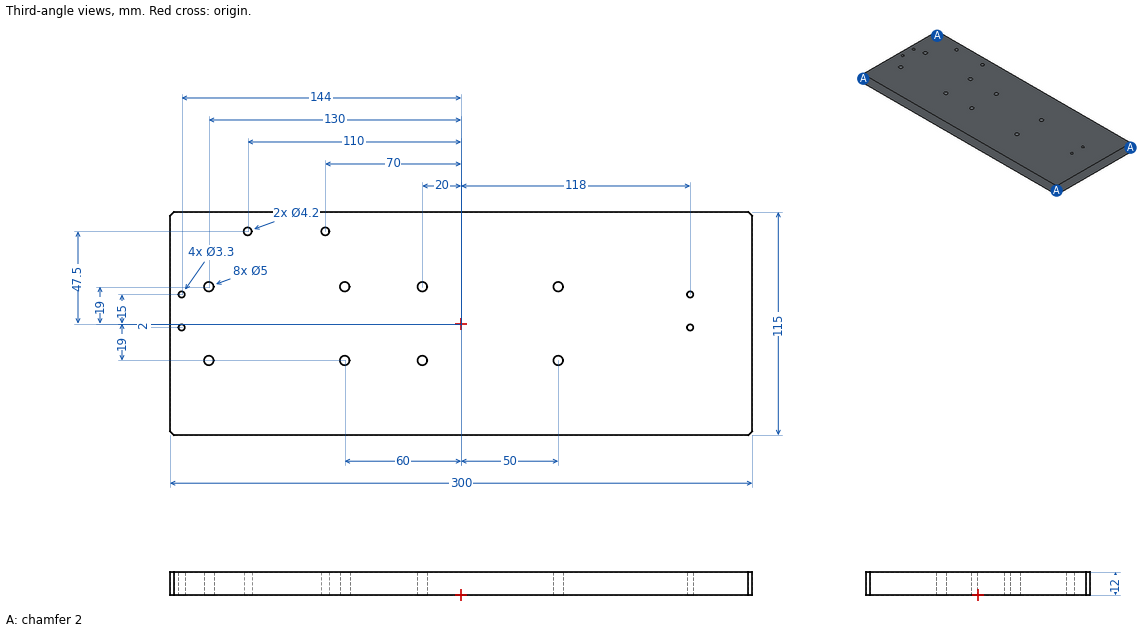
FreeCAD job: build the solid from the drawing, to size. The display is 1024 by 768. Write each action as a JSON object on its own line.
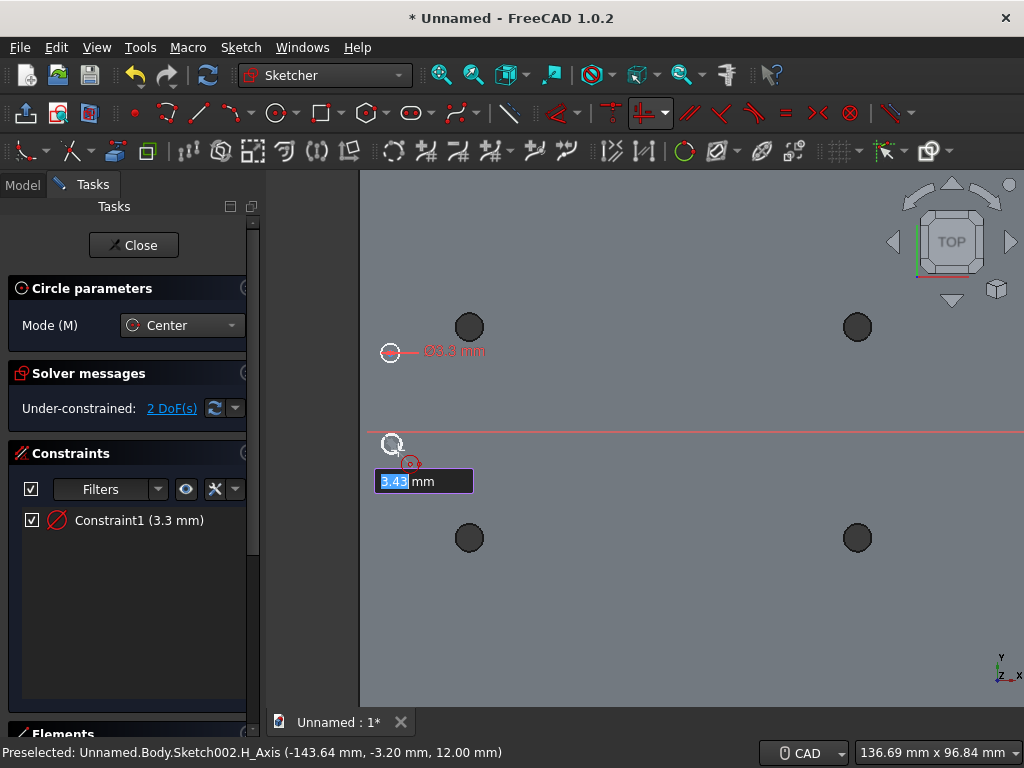
{"action": "type", "text": "3.3"}
{"action": "key", "text": "Return"}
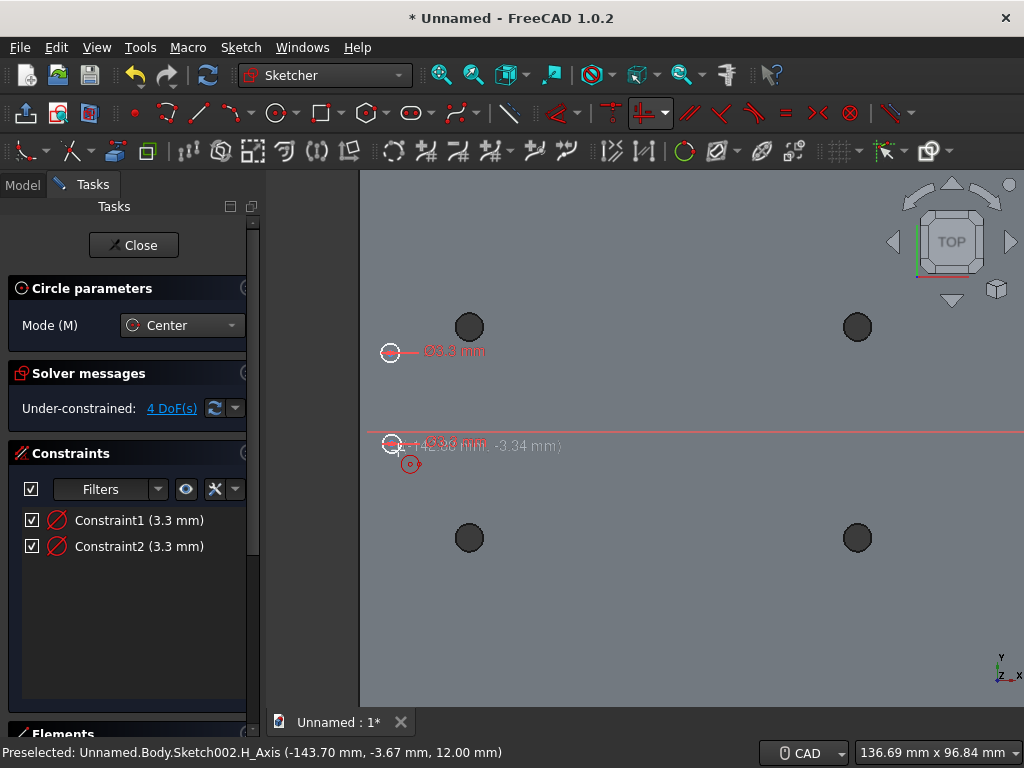
{"action": "scroll", "coordinate": [399, 452], "scroll_direction": "down", "scroll_amount": 7}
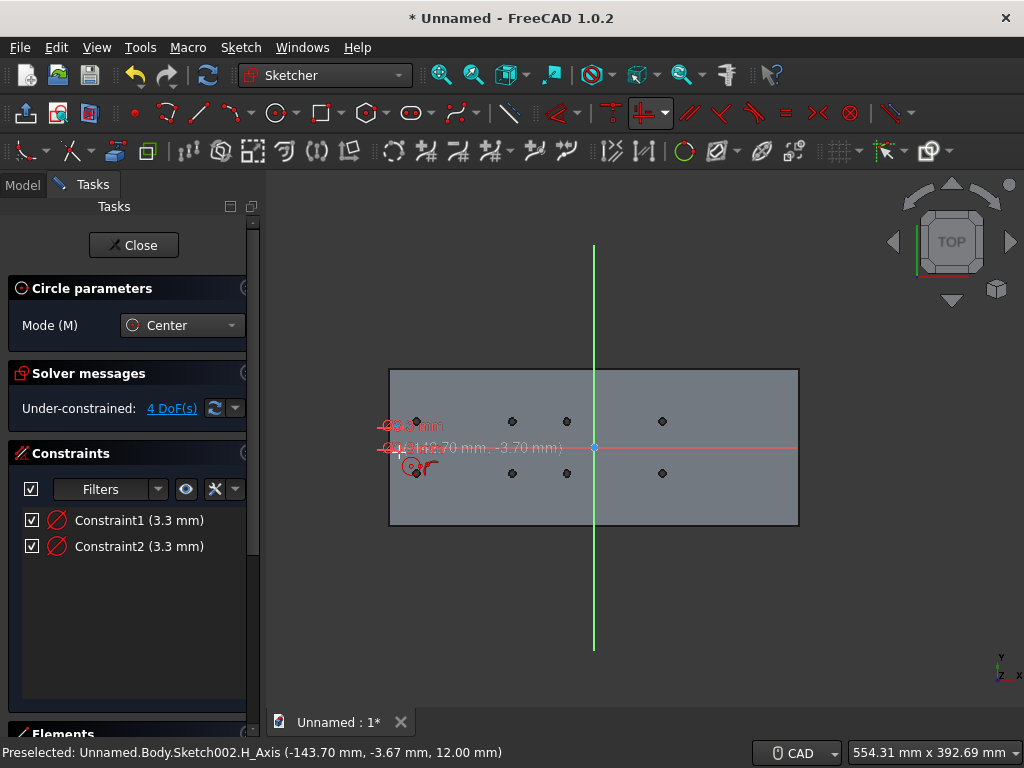
{"action": "scroll", "coordinate": [756, 427], "scroll_direction": "up", "scroll_amount": 12}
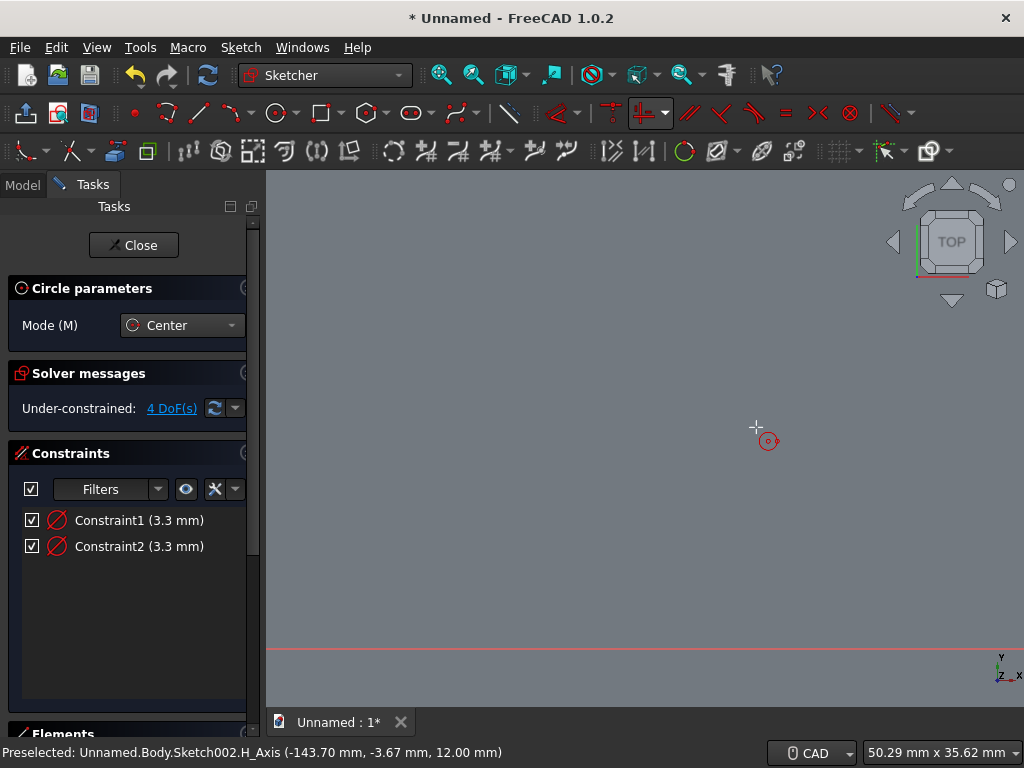
{"action": "scroll", "coordinate": [757, 427], "scroll_direction": "down", "scroll_amount": 12}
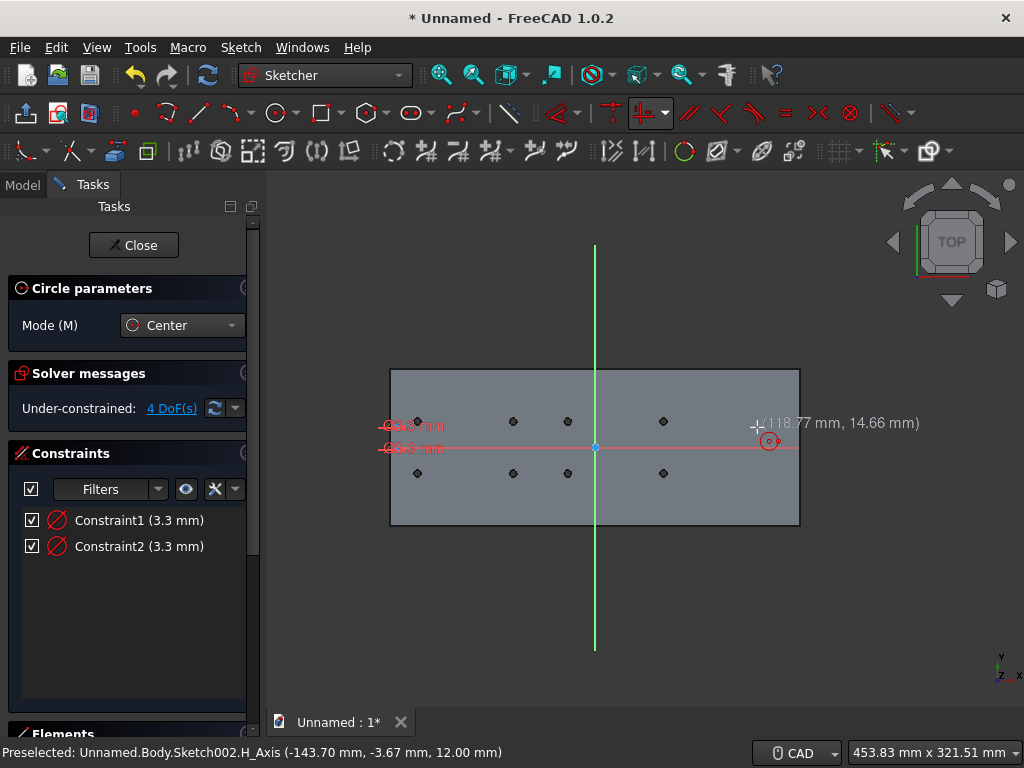
{"action": "left_click", "coordinate": [757, 427]}
{"action": "mouse_move", "coordinate": [758, 425]}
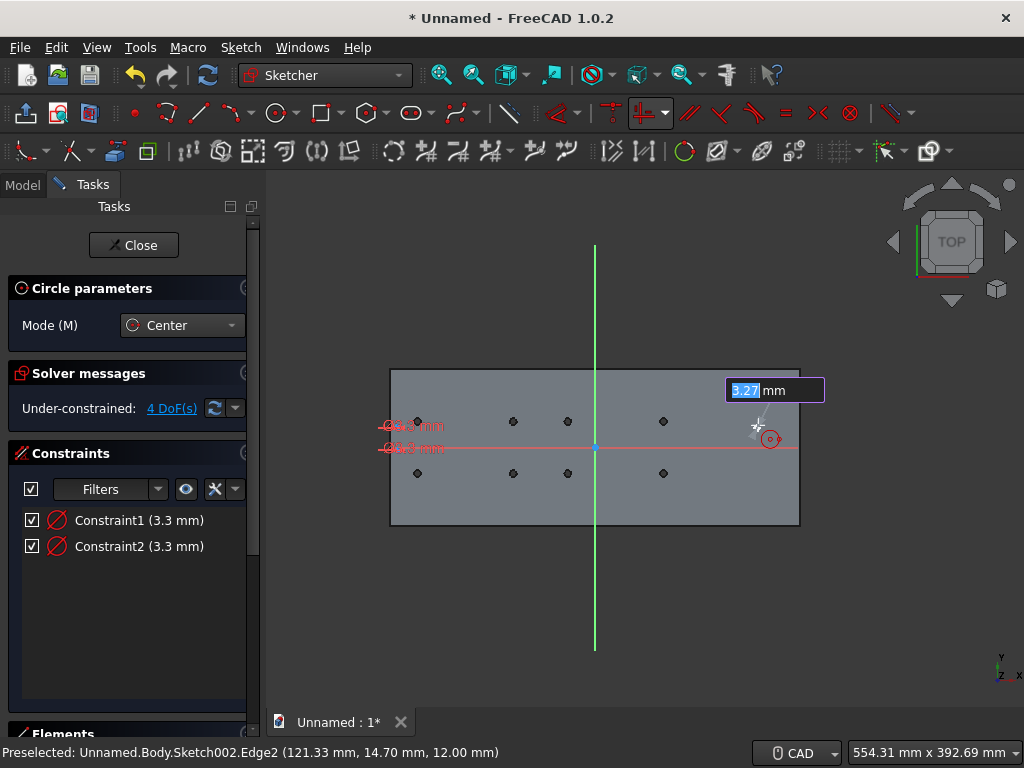
{"action": "type", "text": "3.3"}
{"action": "key", "text": "Return"}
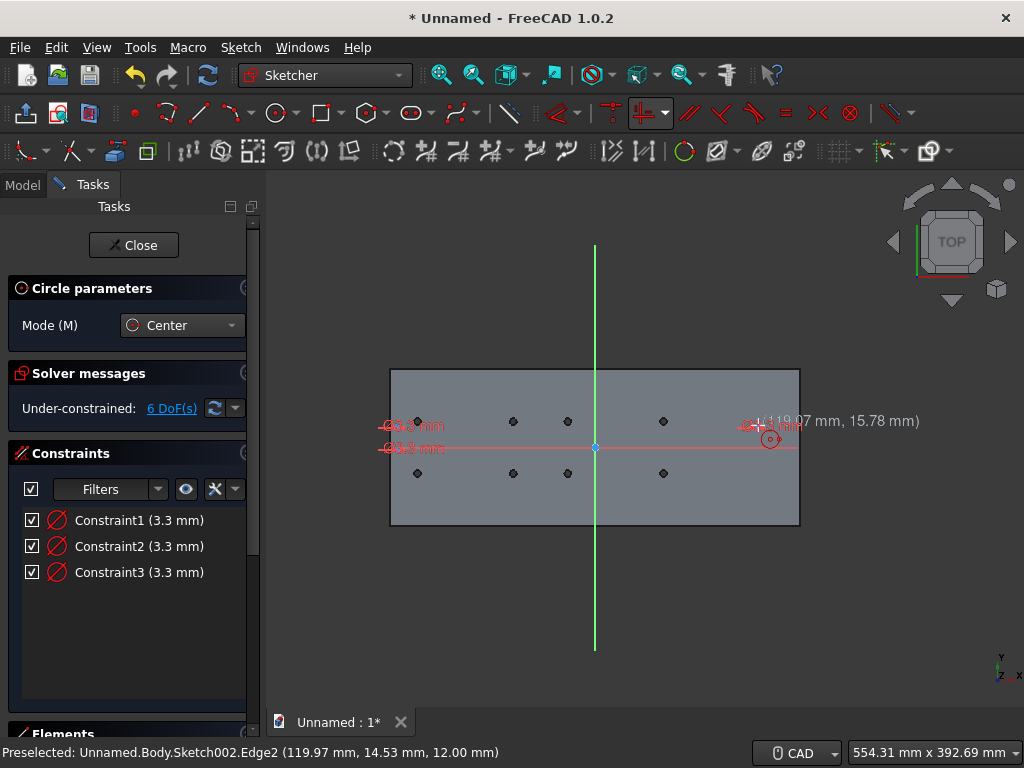
{"action": "scroll", "coordinate": [757, 450], "scroll_direction": "up", "scroll_amount": 12}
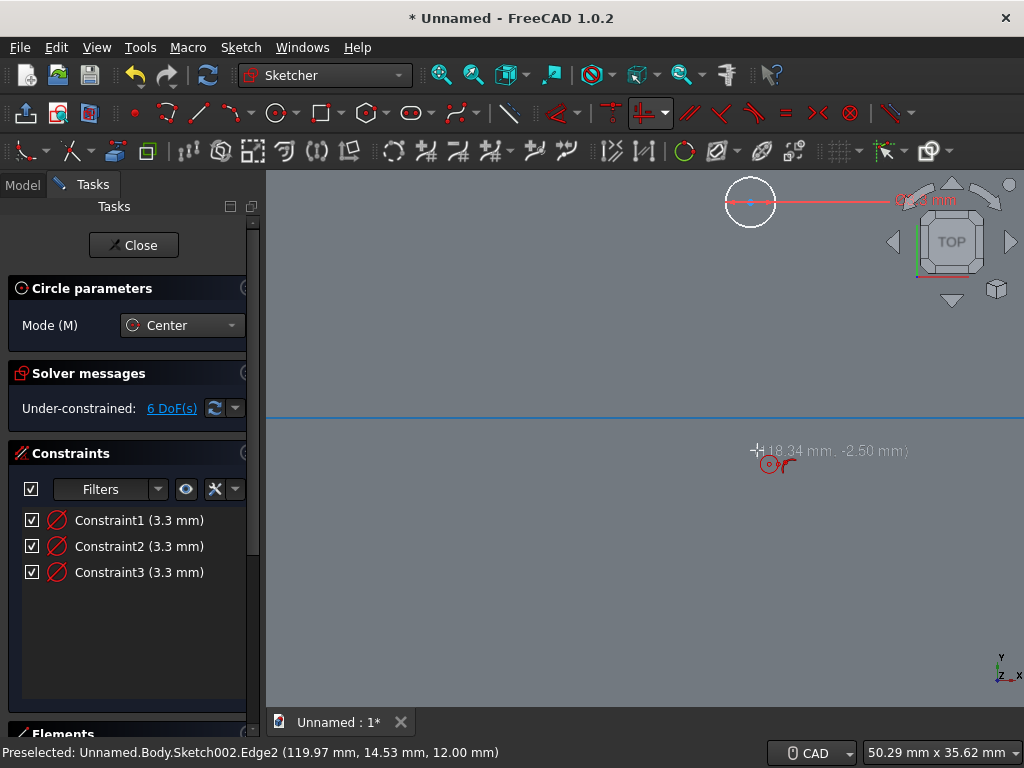
{"action": "left_click", "coordinate": [745, 448]}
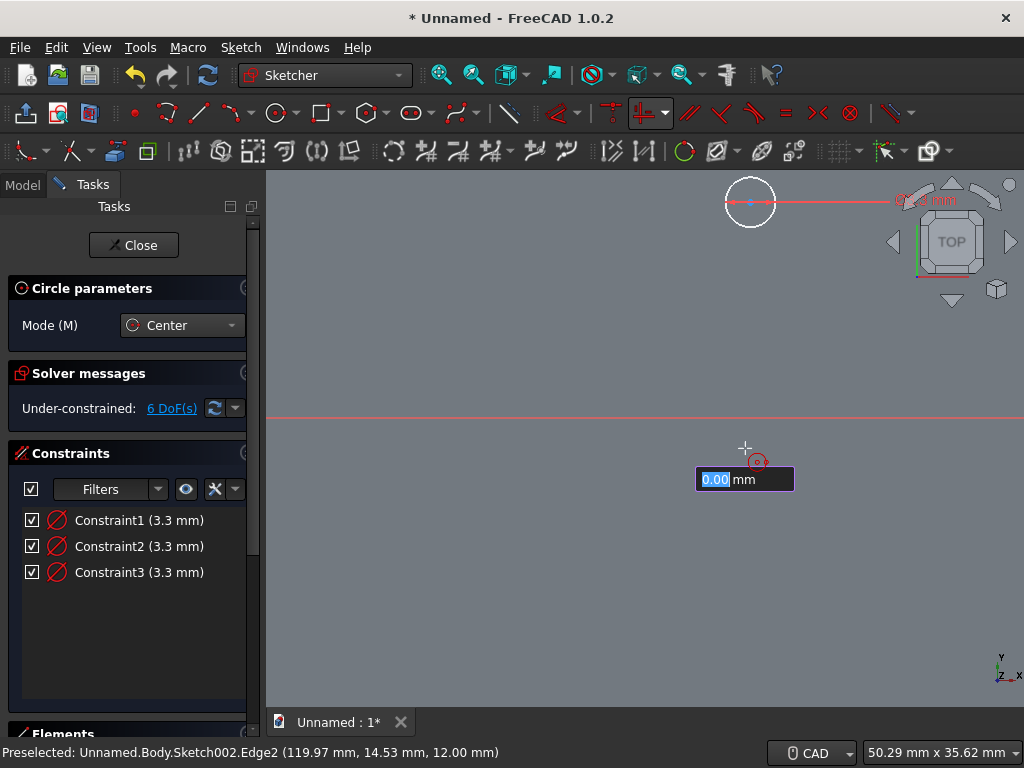
{"action": "scroll", "coordinate": [757, 450], "scroll_direction": "down", "scroll_amount": 12}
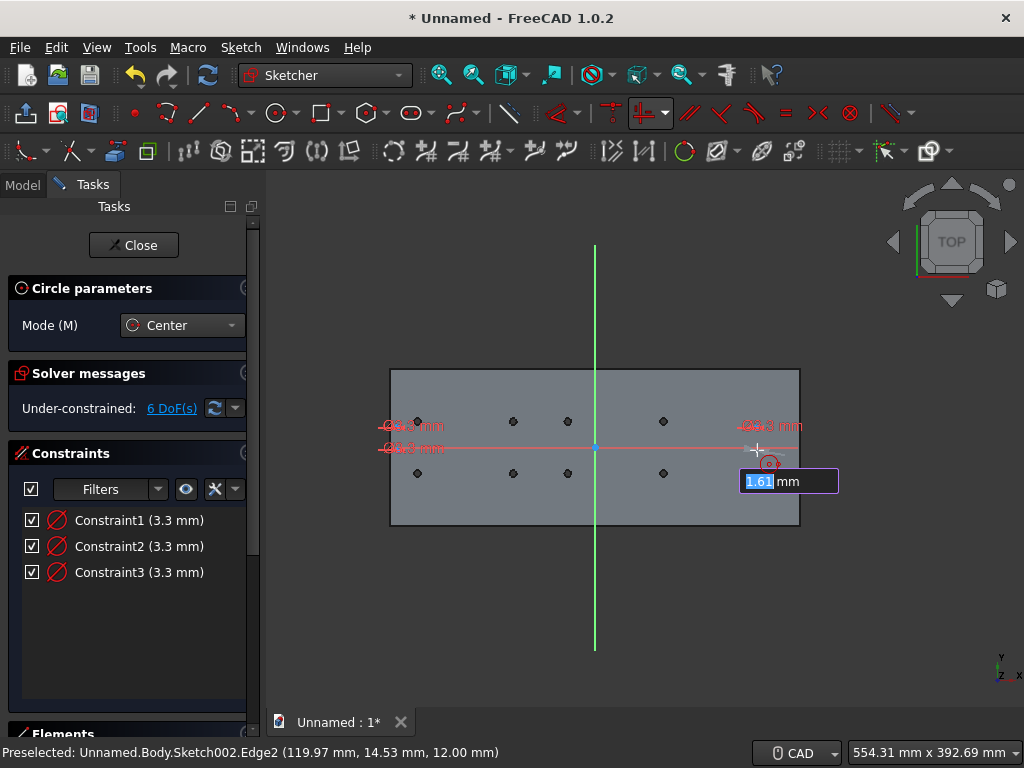
{"action": "scroll", "coordinate": [758, 452], "scroll_direction": "up", "scroll_amount": 7}
{"action": "mouse_move", "coordinate": [757, 450]}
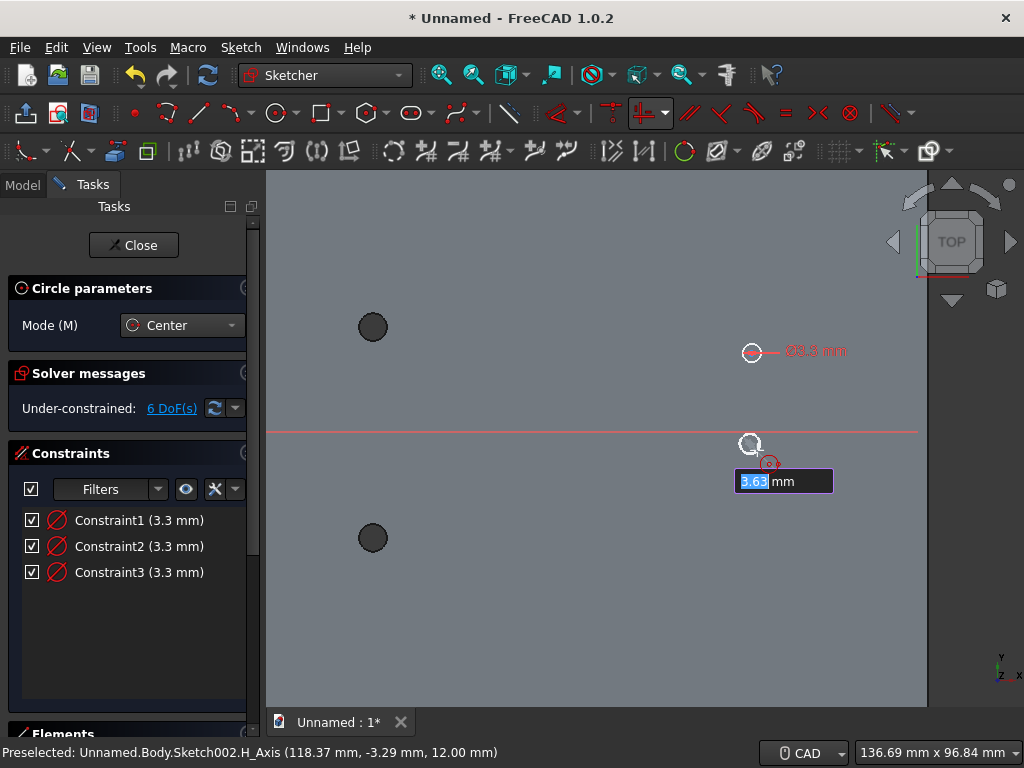
{"action": "type", "text": "3.3"}
{"action": "key", "text": "Return"}
{"action": "key", "text": "Escape"}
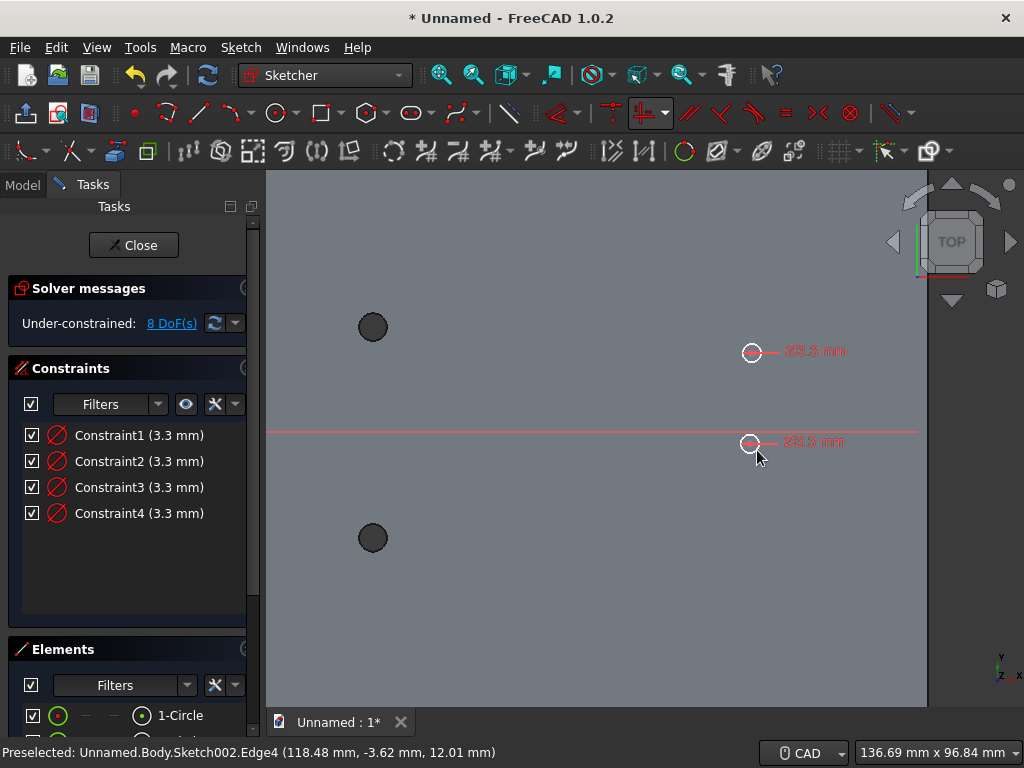
{"action": "scroll", "coordinate": [757, 452], "scroll_direction": "down", "scroll_amount": 7}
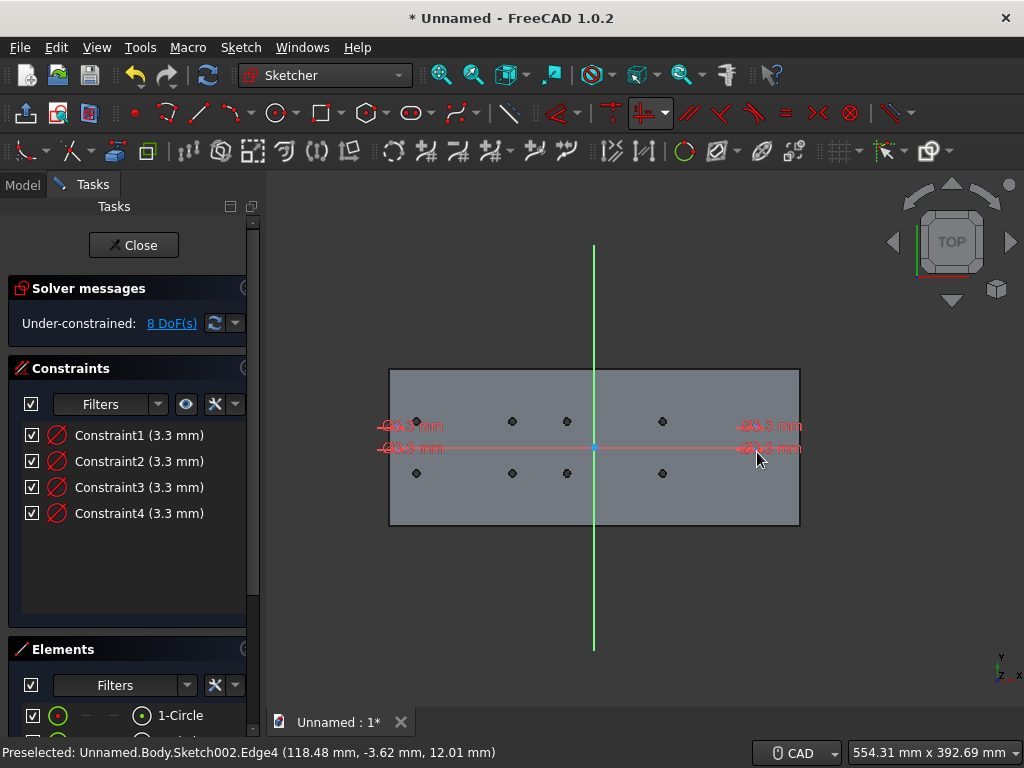
{"action": "left_click", "coordinate": [397, 428]}